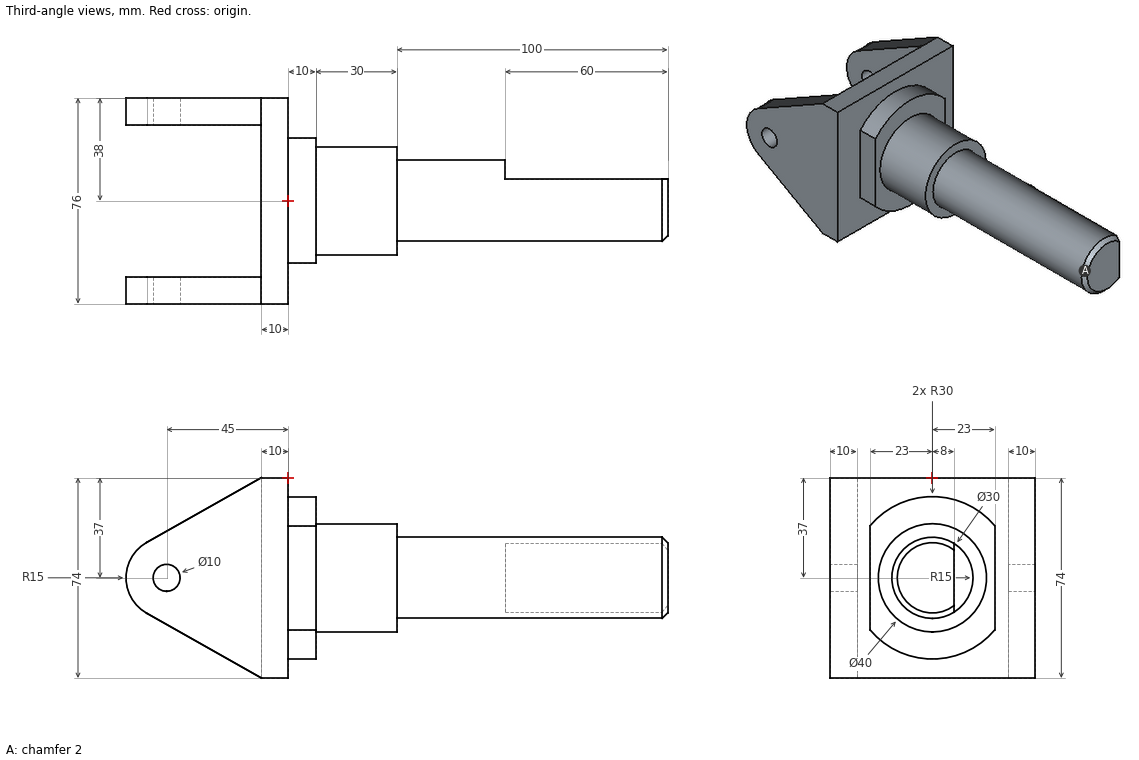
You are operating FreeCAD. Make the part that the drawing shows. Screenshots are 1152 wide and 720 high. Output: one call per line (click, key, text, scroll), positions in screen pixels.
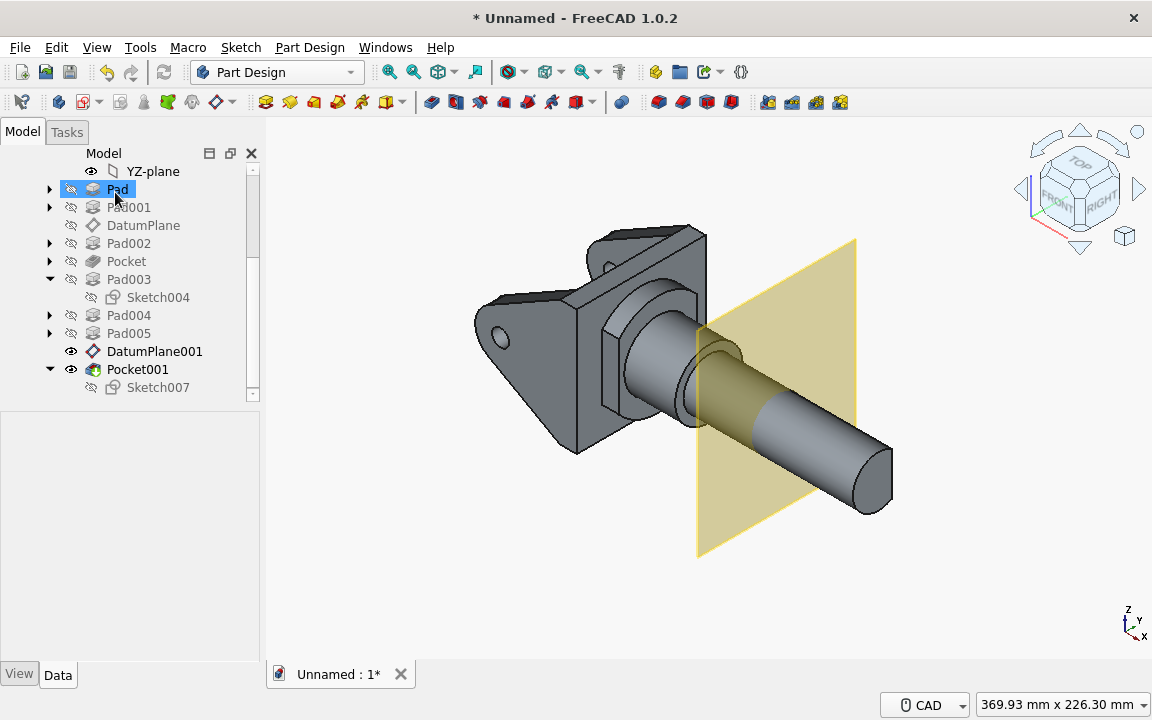
click(116, 351)
key(space)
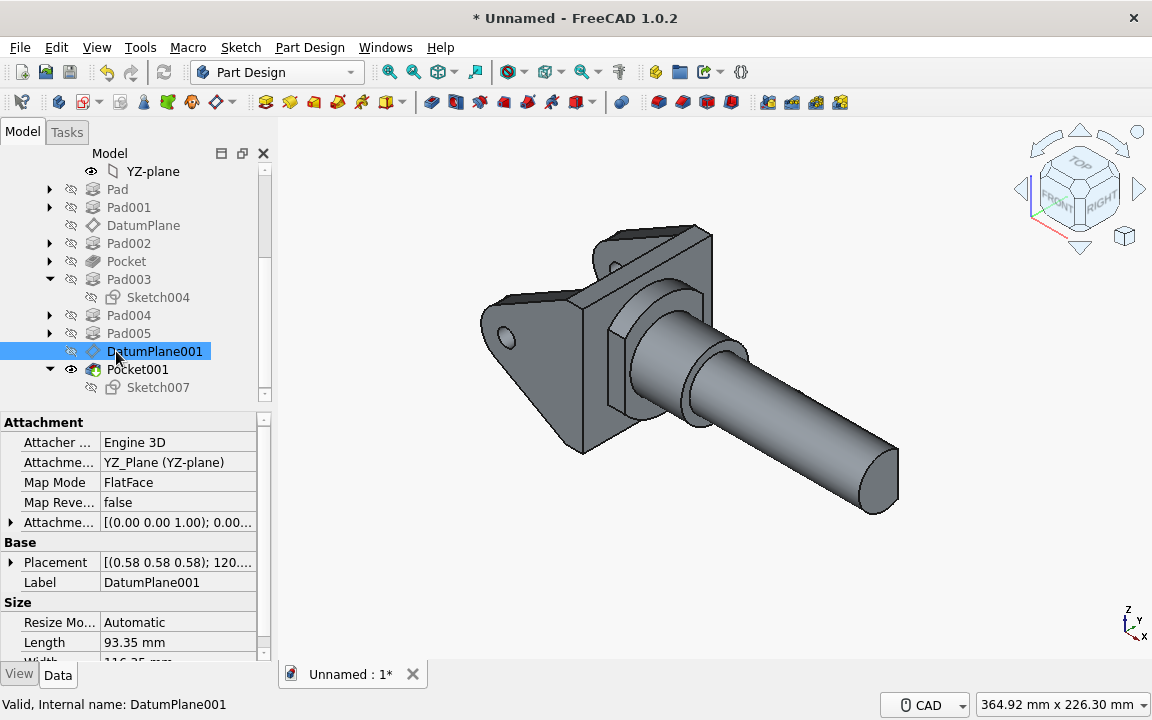
click(859, 495)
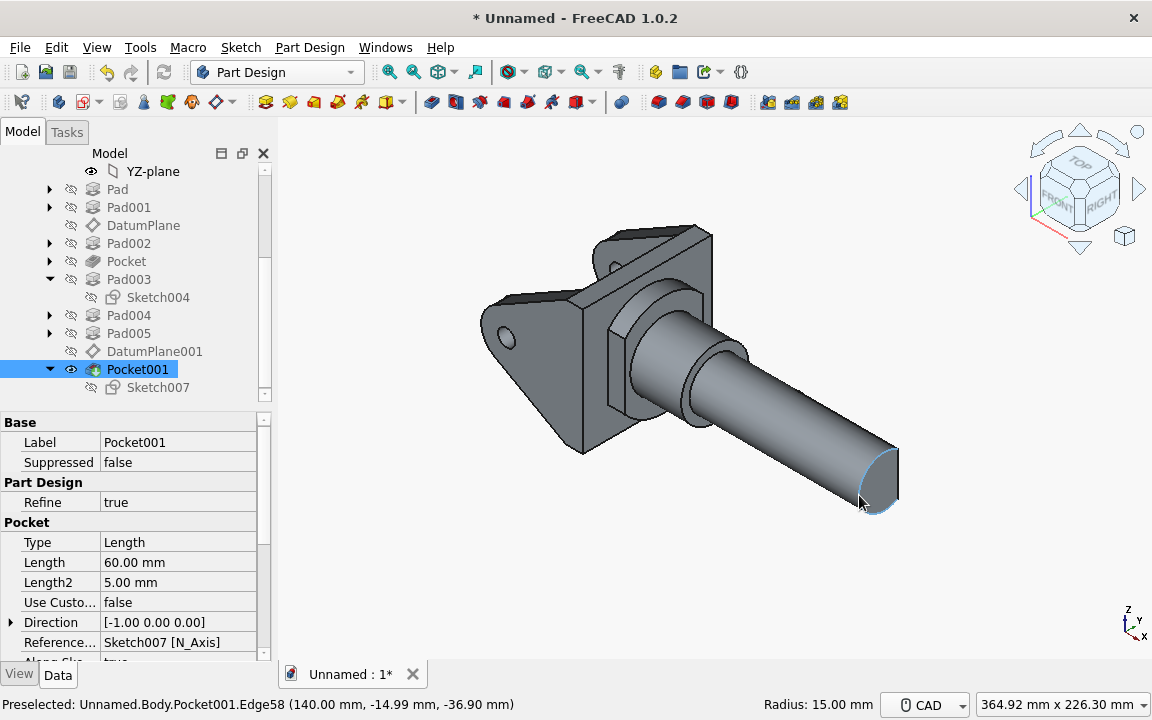
click(684, 102)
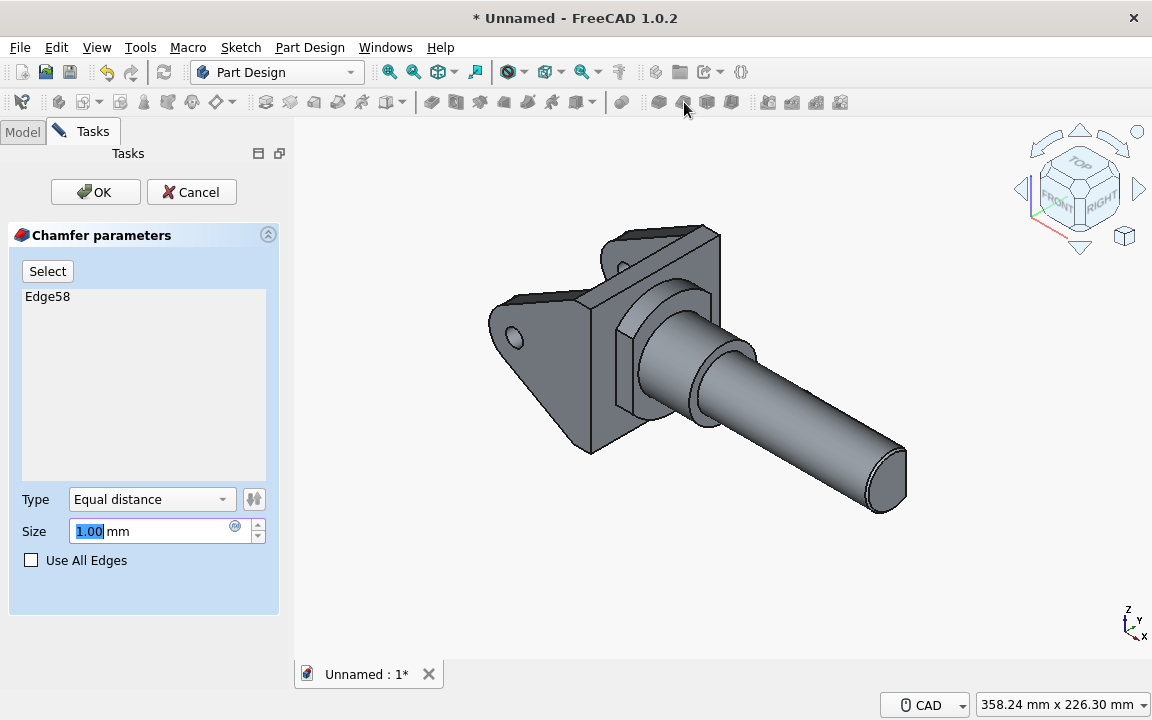
text(2)
key(Tab)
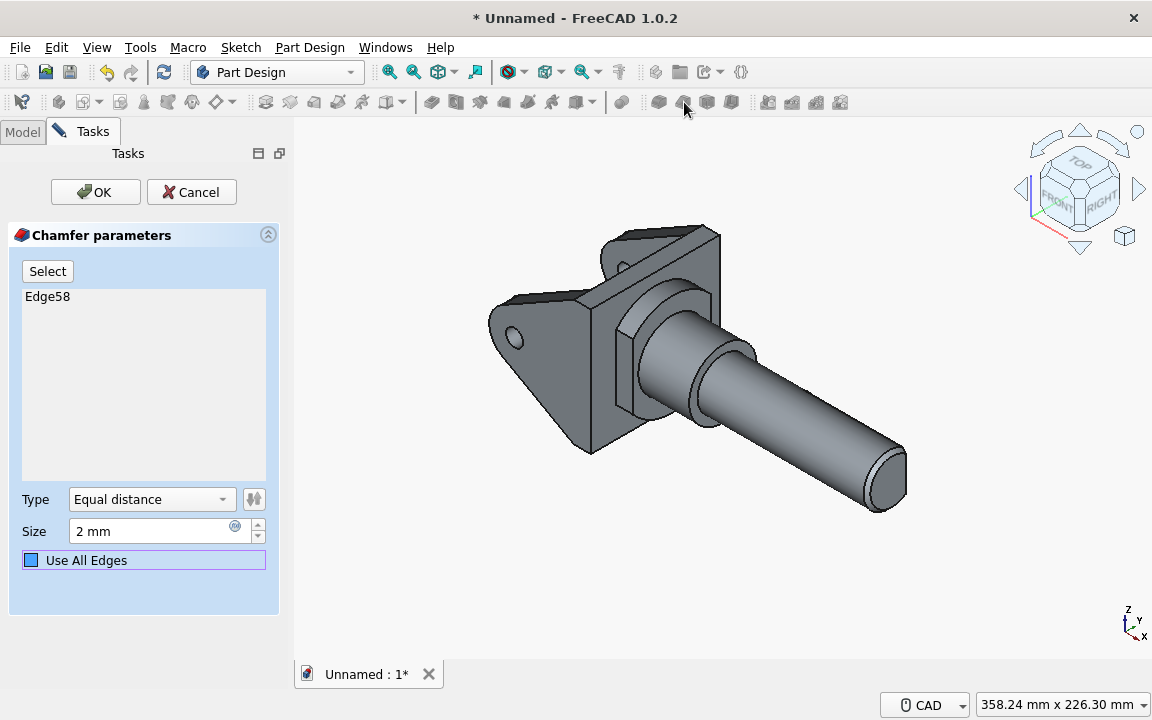
click(96, 192)